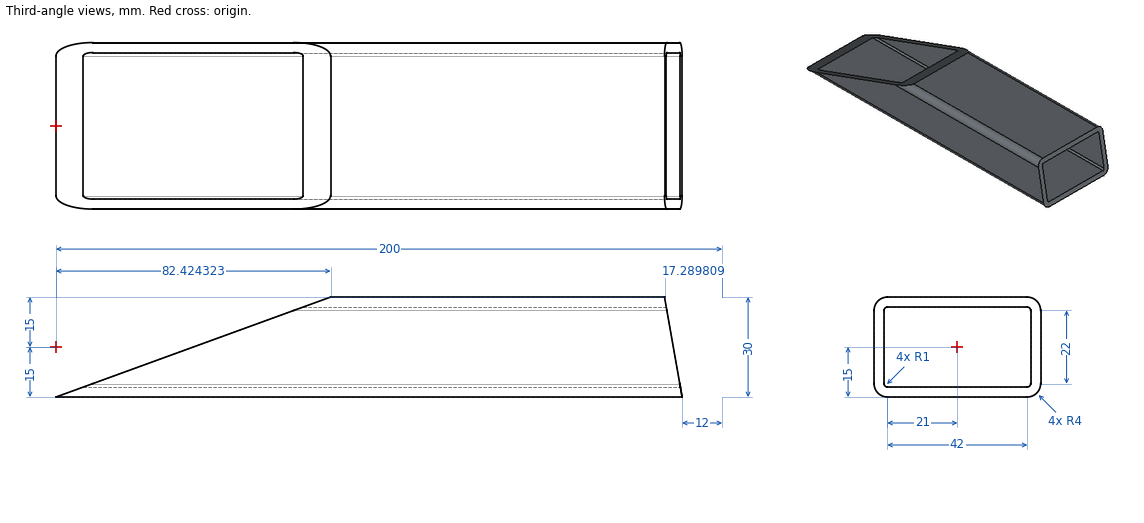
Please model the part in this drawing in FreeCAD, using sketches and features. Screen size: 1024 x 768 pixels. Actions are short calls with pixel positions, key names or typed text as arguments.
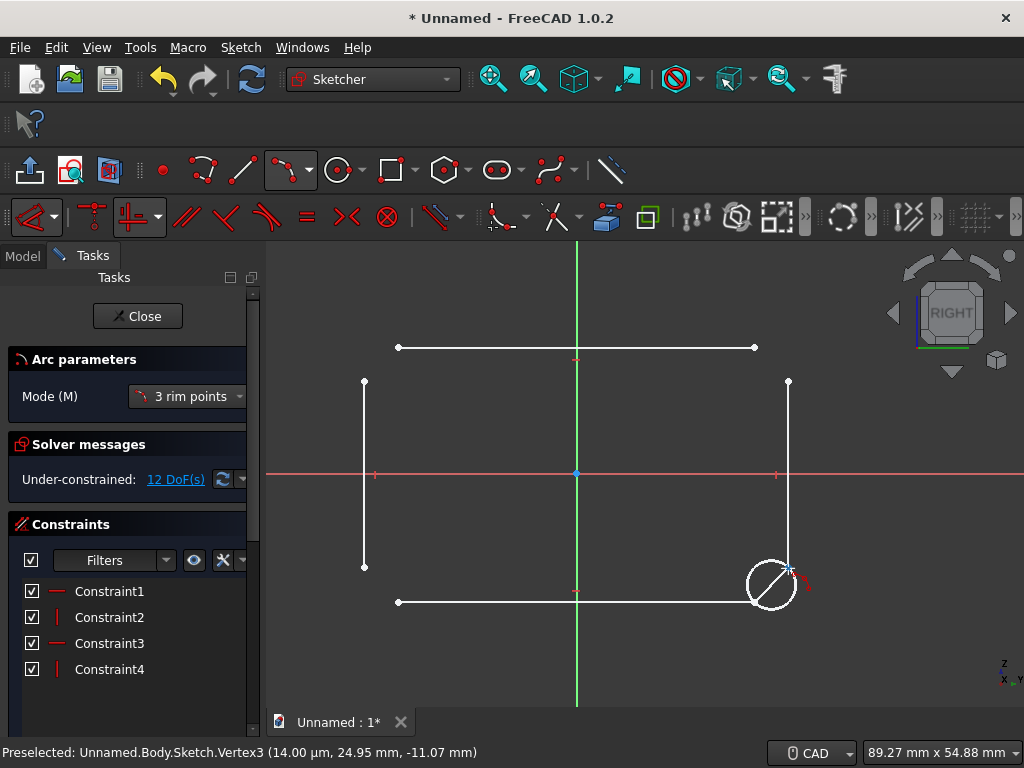
scroll(779, 591, up, 3)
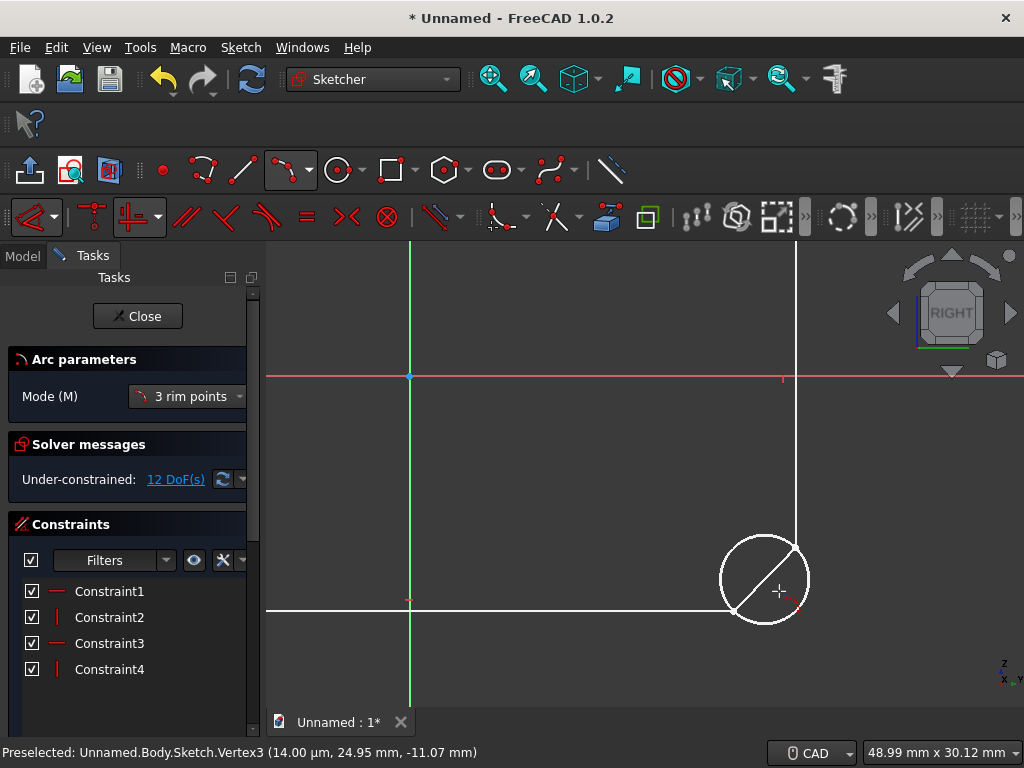
click(778, 590)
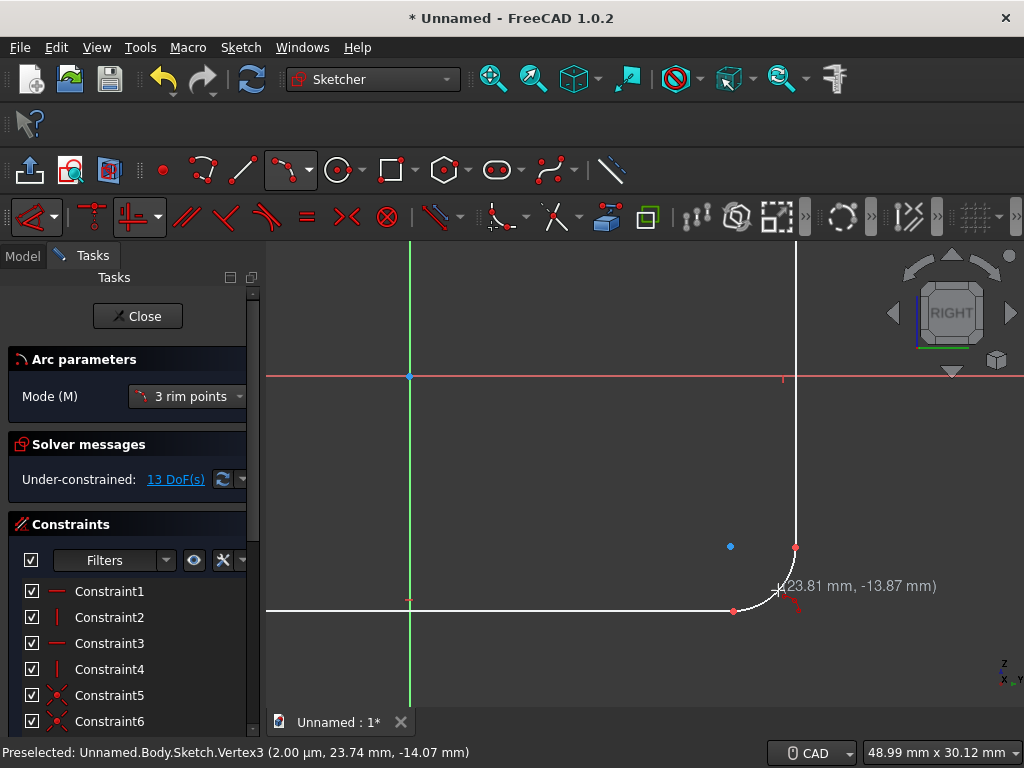
scroll(780, 593, down, 3)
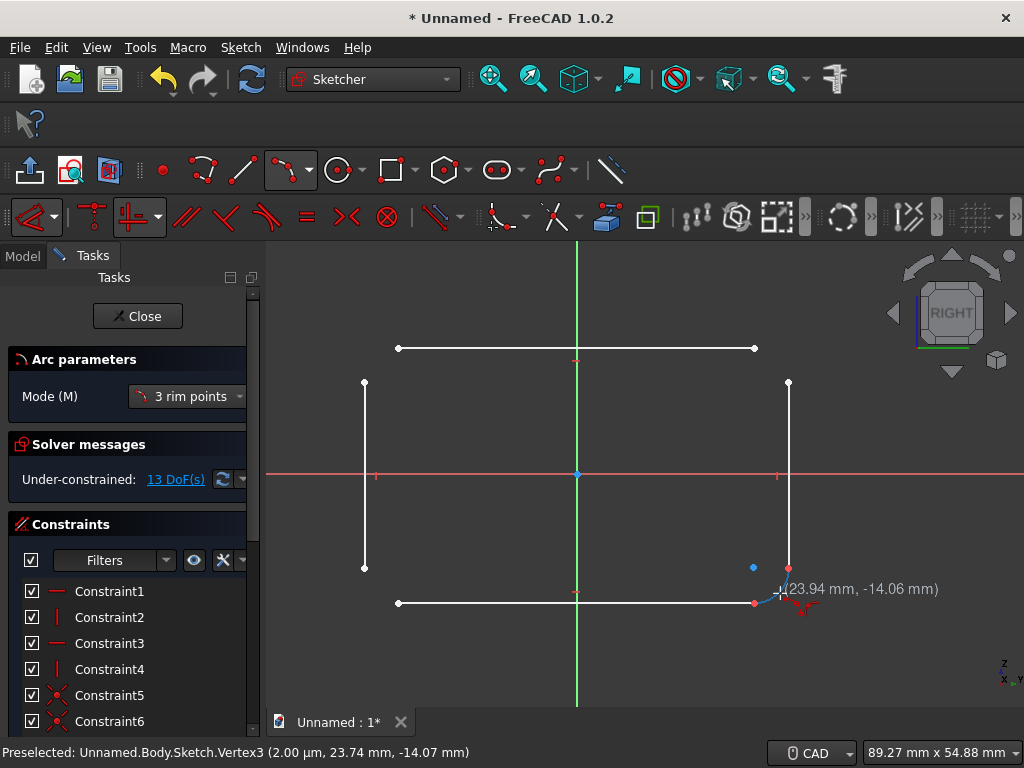
click(789, 382)
click(755, 348)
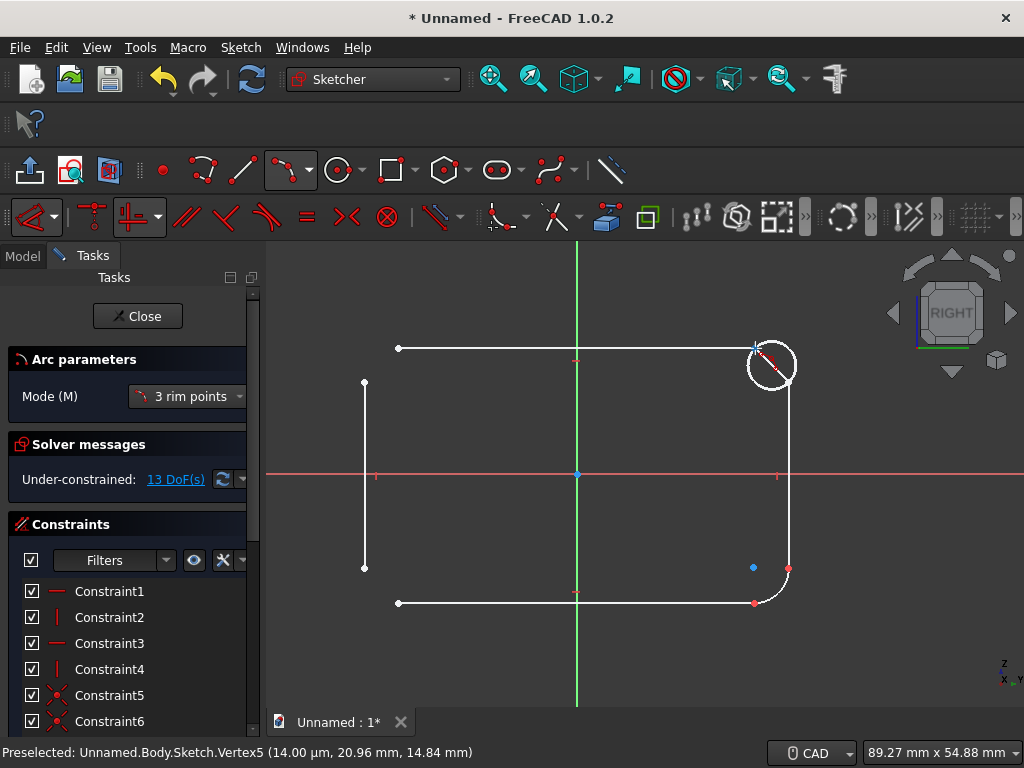
scroll(779, 357, up, 3)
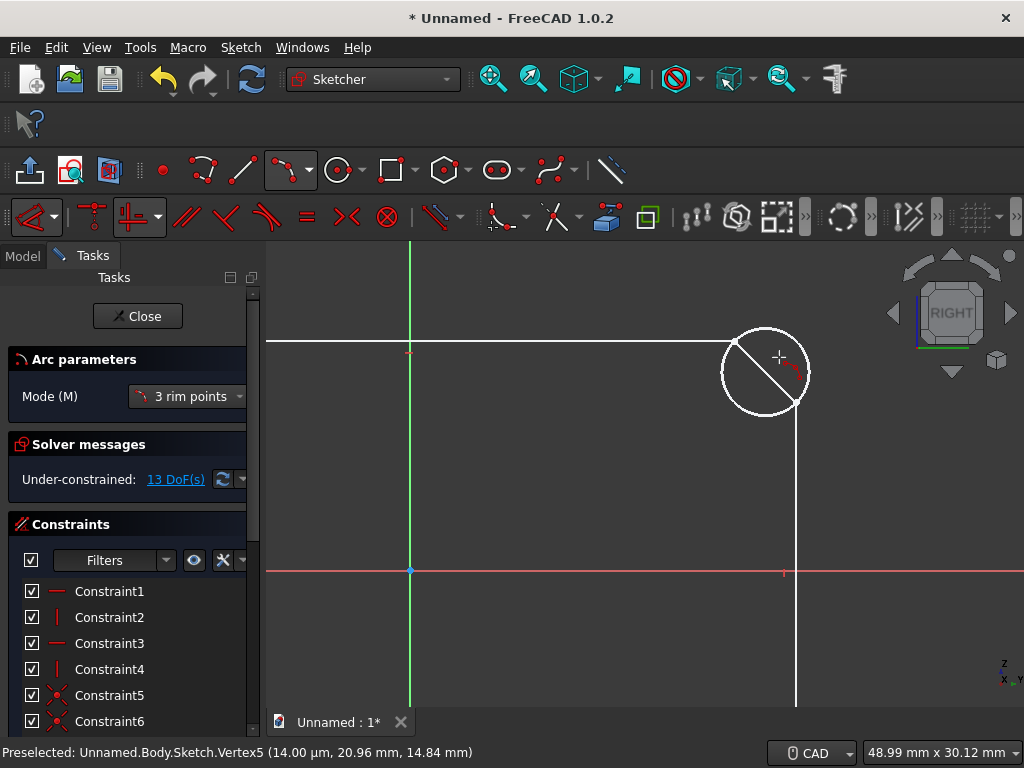
click(779, 357)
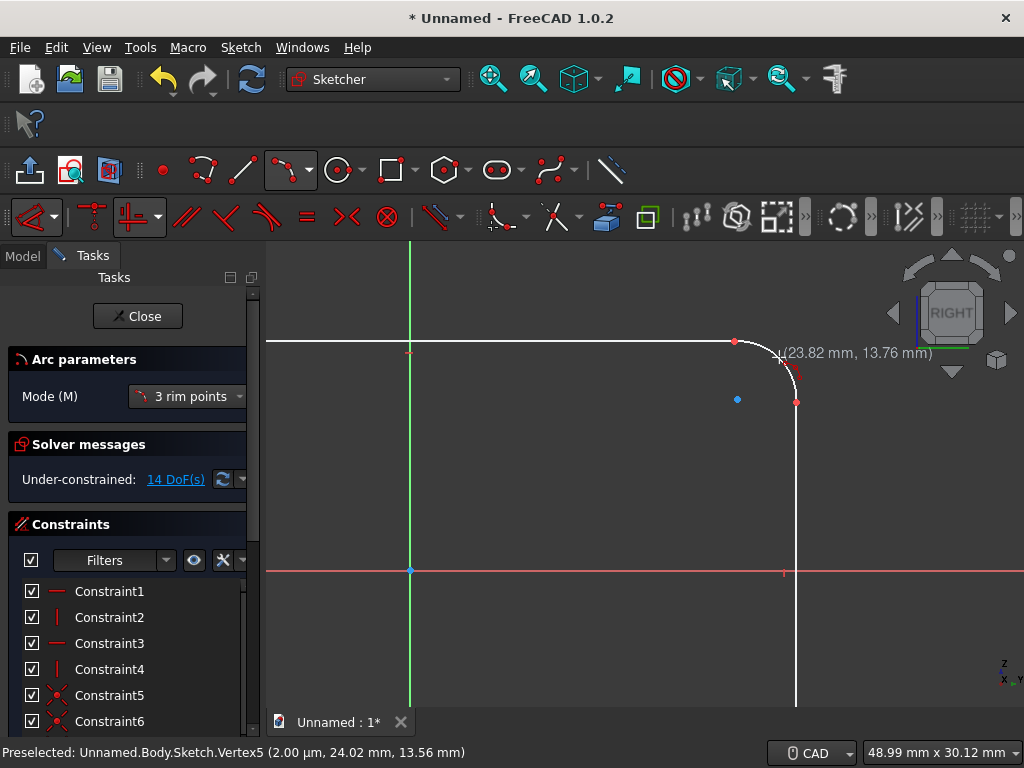
scroll(779, 356, down, 3)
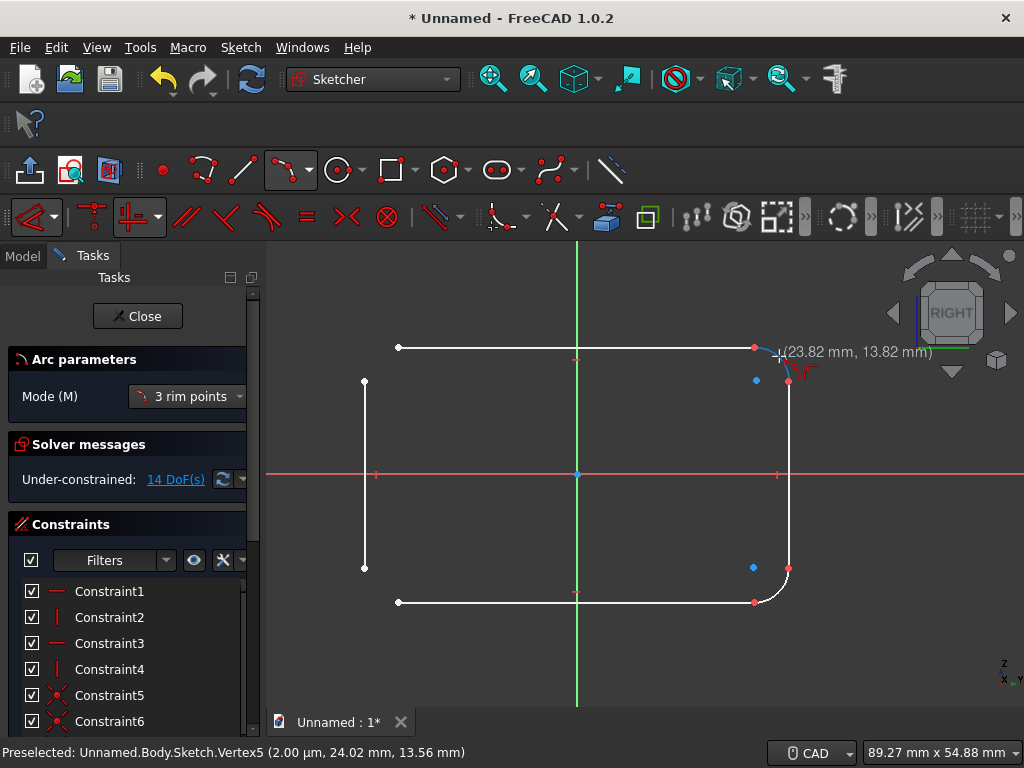
click(399, 348)
click(365, 382)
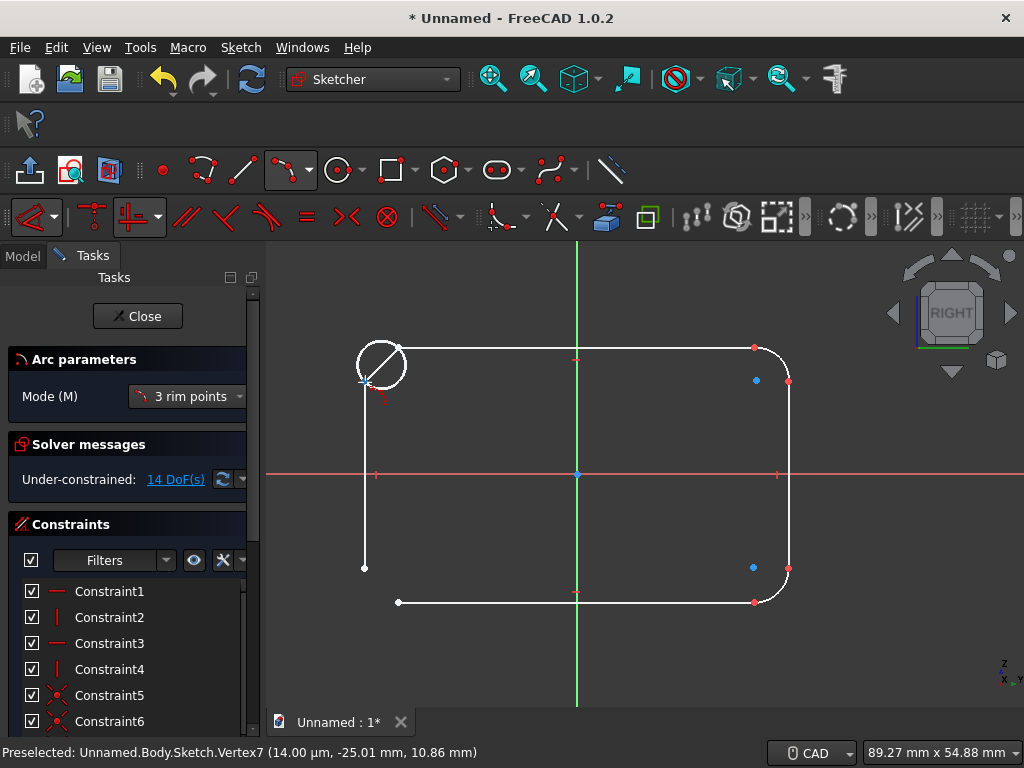
scroll(375, 357, up, 3)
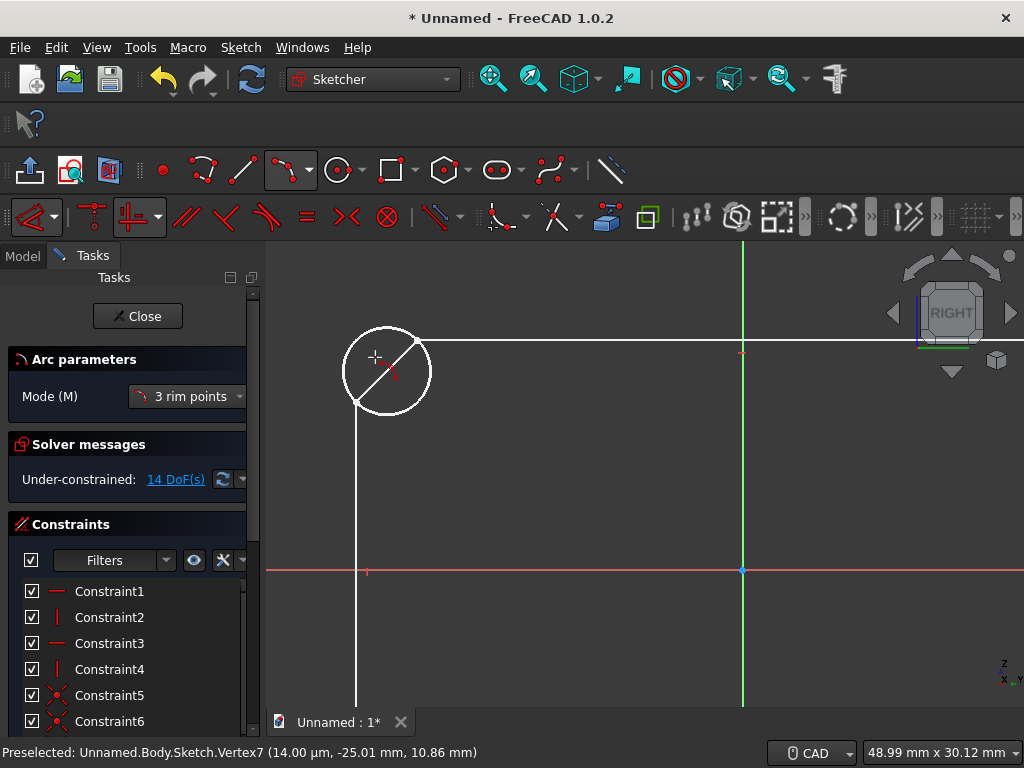
click(374, 356)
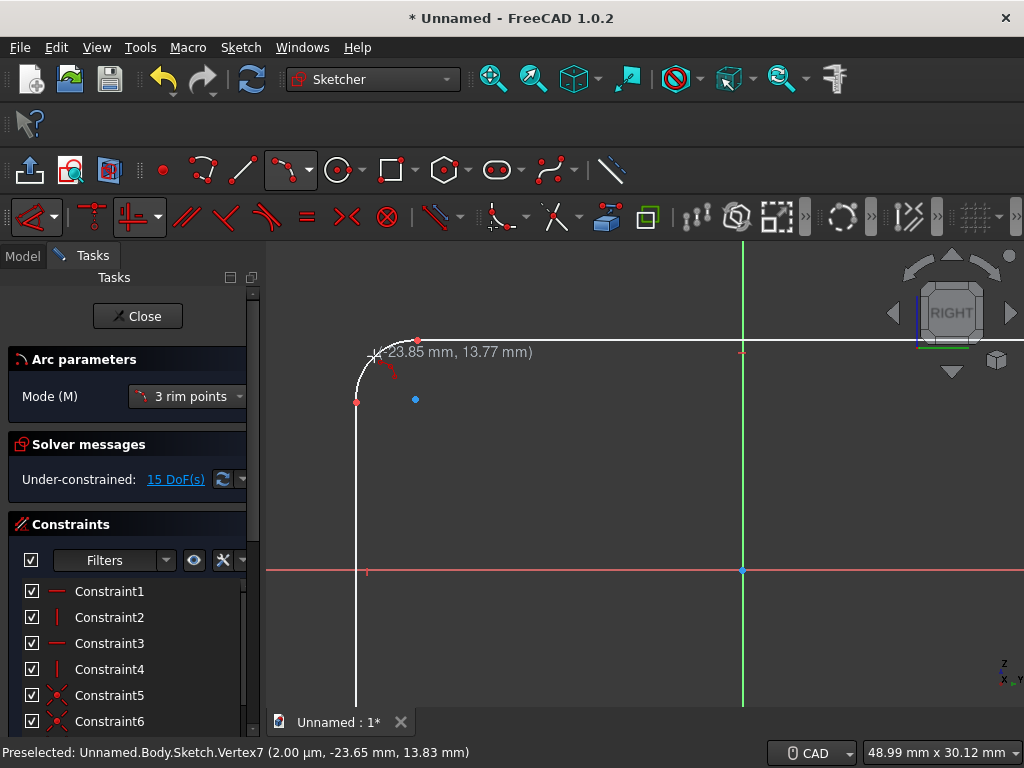
scroll(374, 357, down, 3)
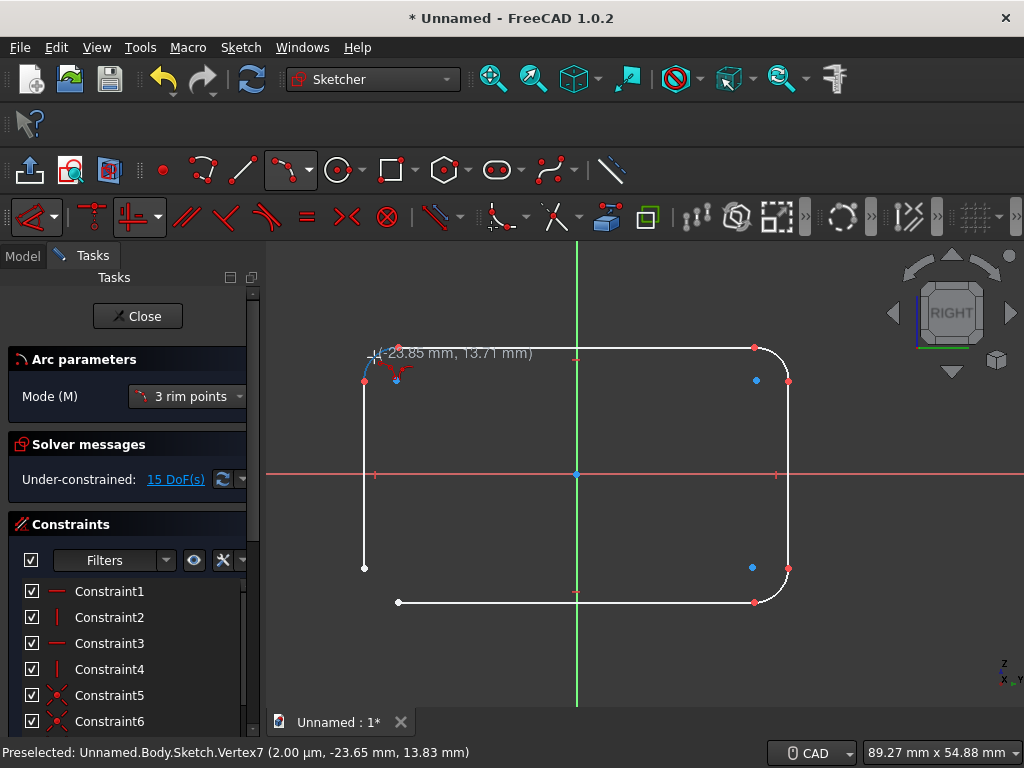
click(364, 568)
click(398, 603)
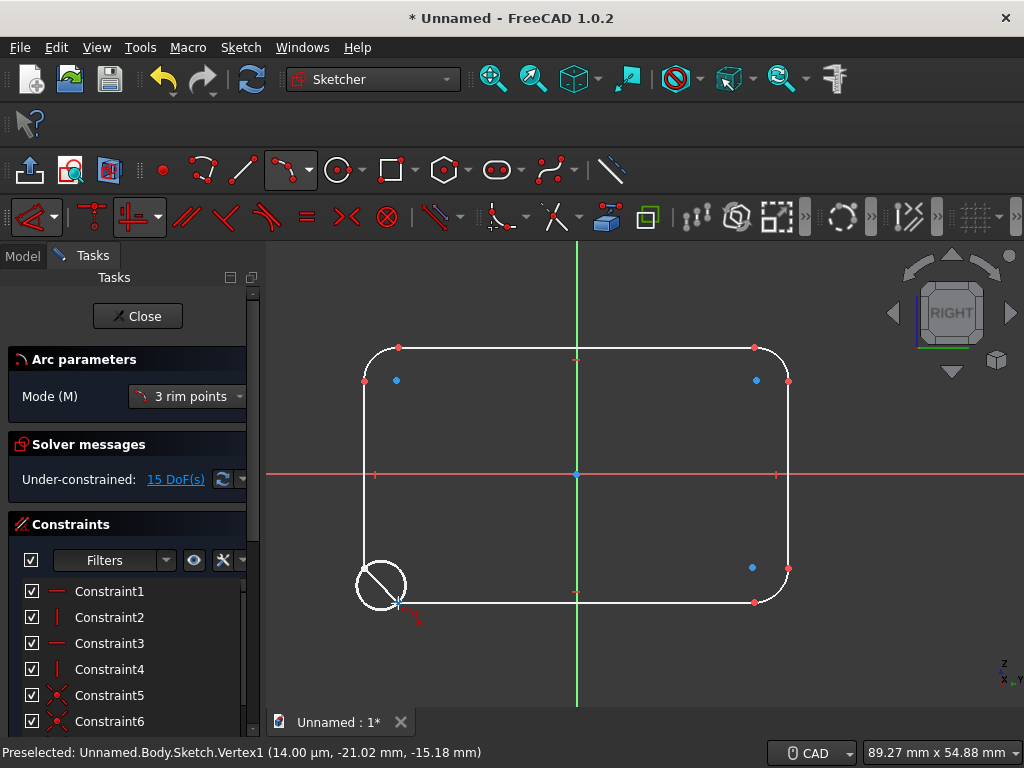
scroll(374, 591, up, 3)